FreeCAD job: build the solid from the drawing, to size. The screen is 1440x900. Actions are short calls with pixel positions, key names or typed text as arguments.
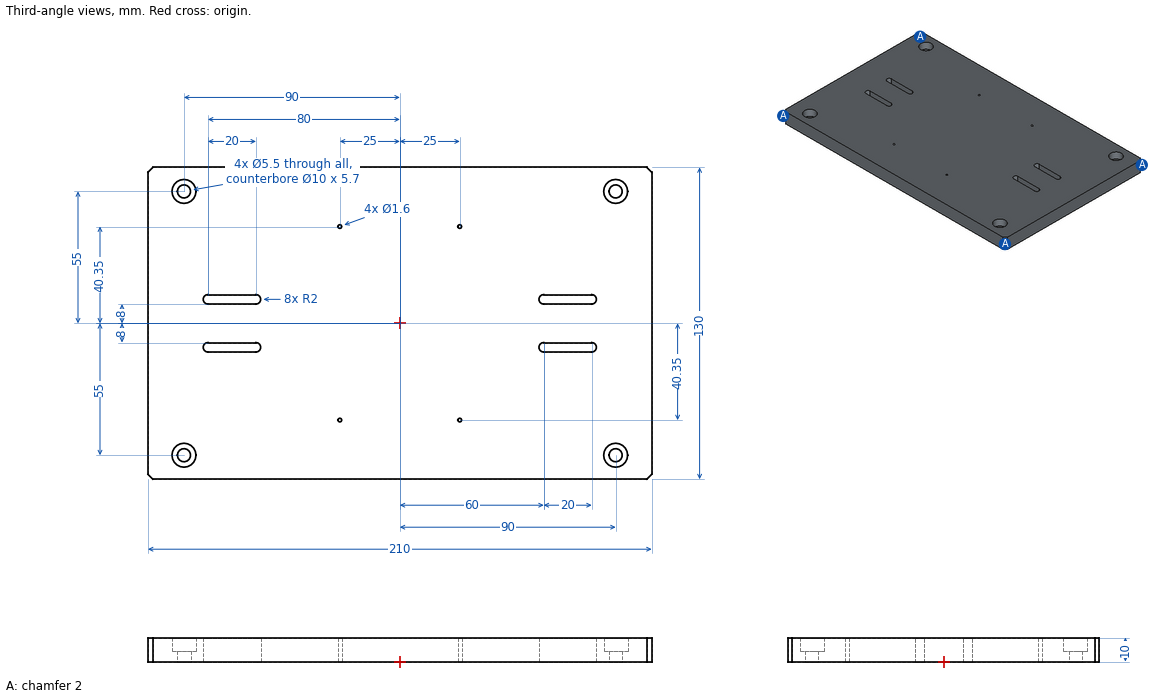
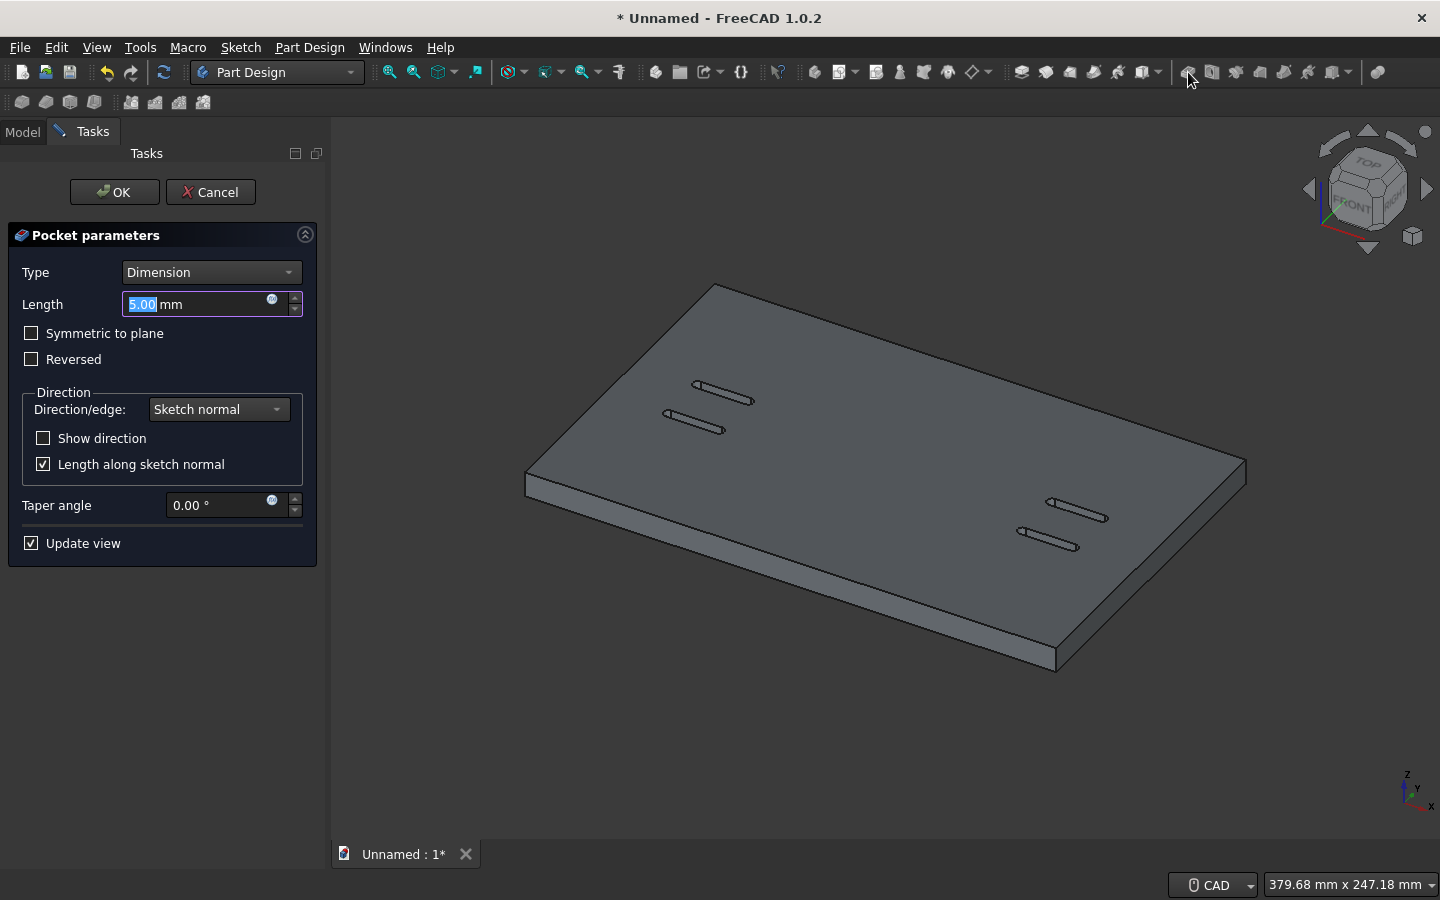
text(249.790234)
key(Tab)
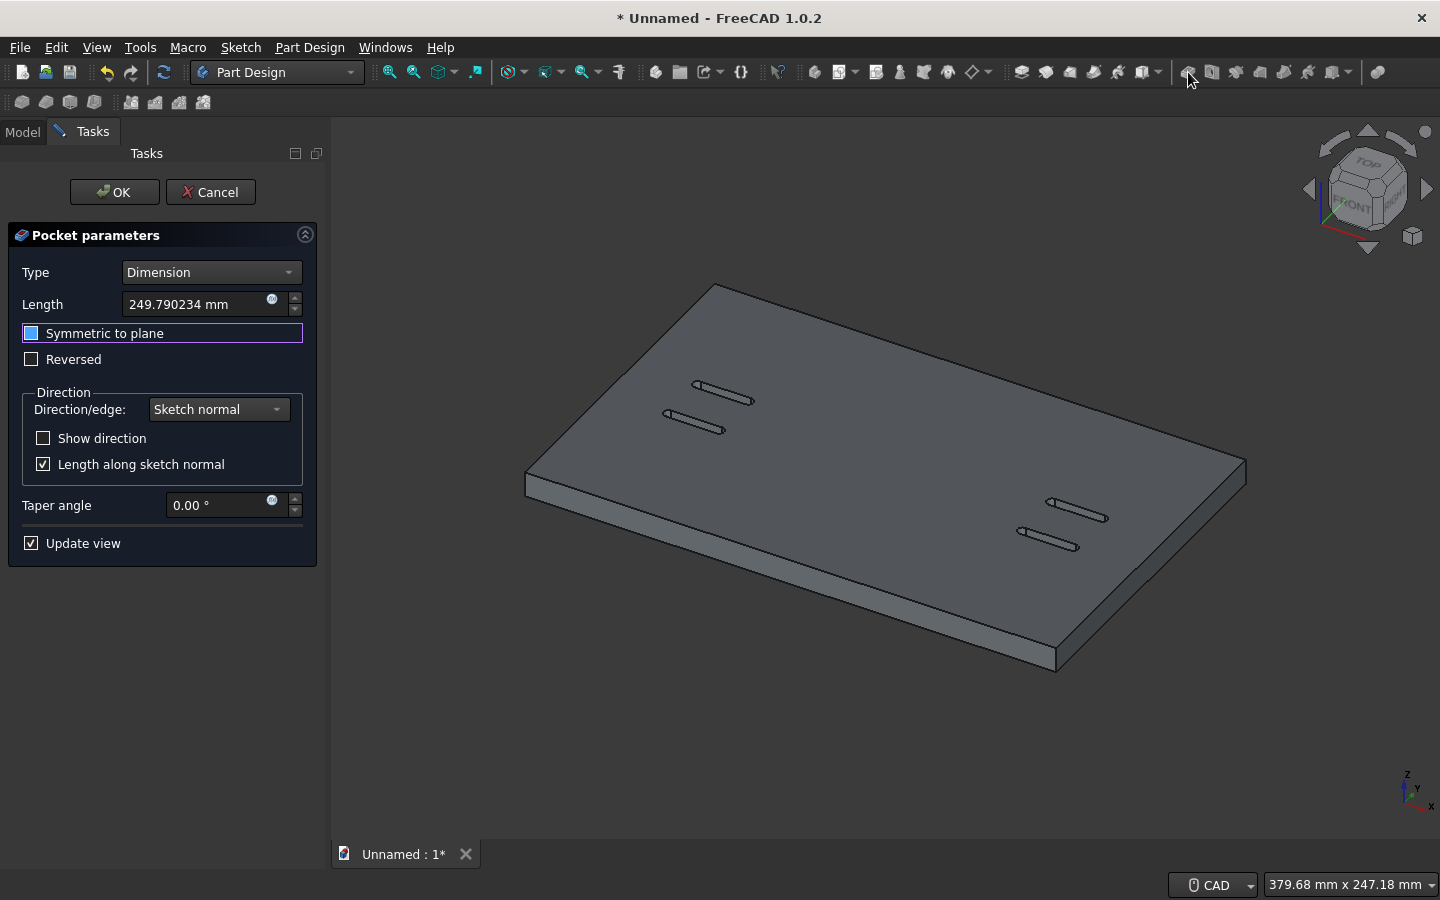
click(30, 333)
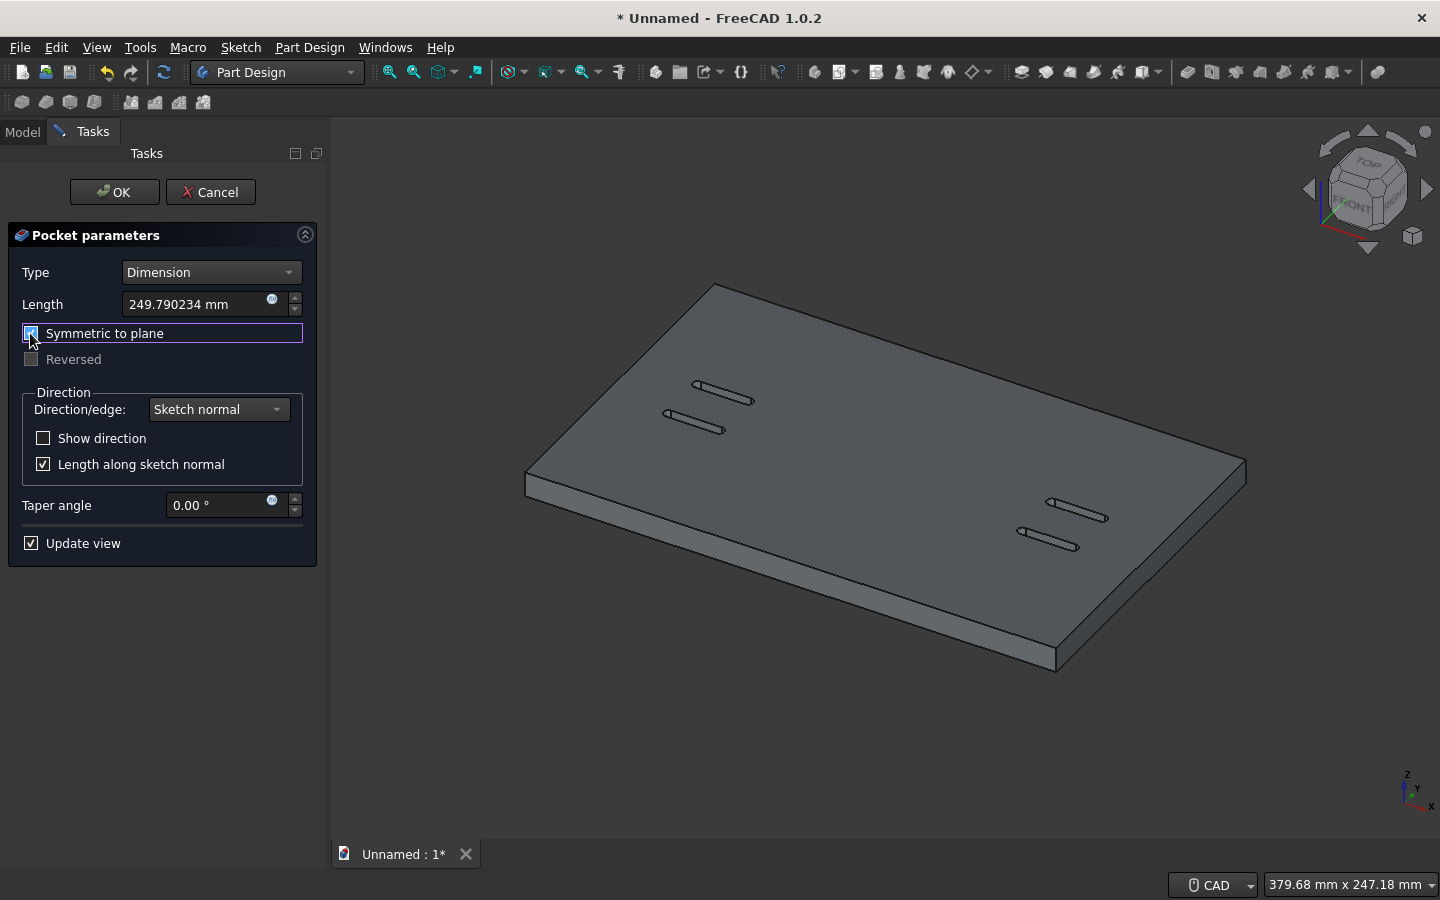
click(115, 192)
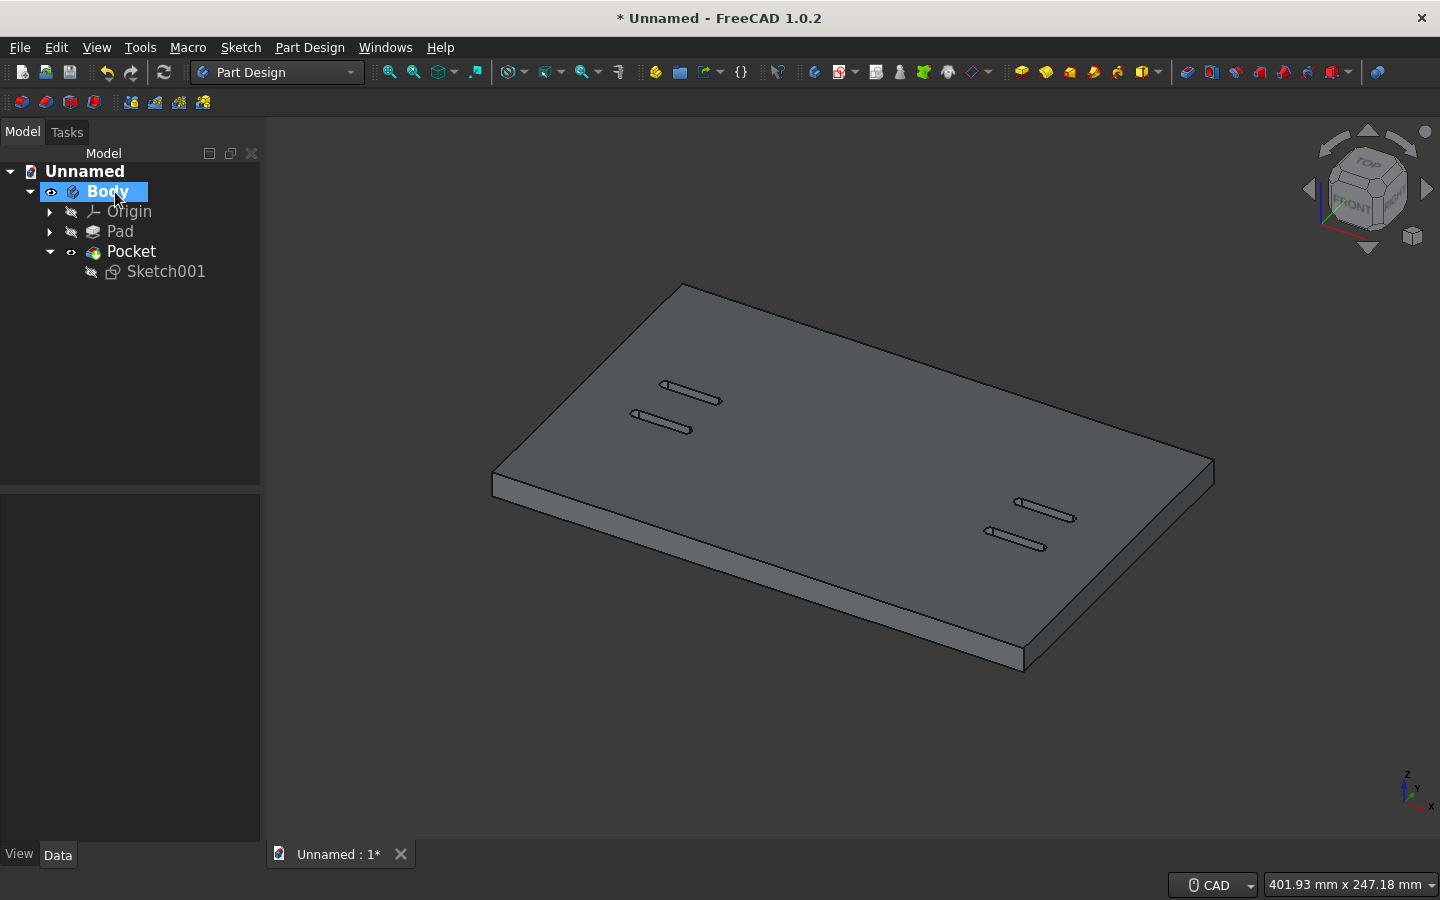
click(853, 465)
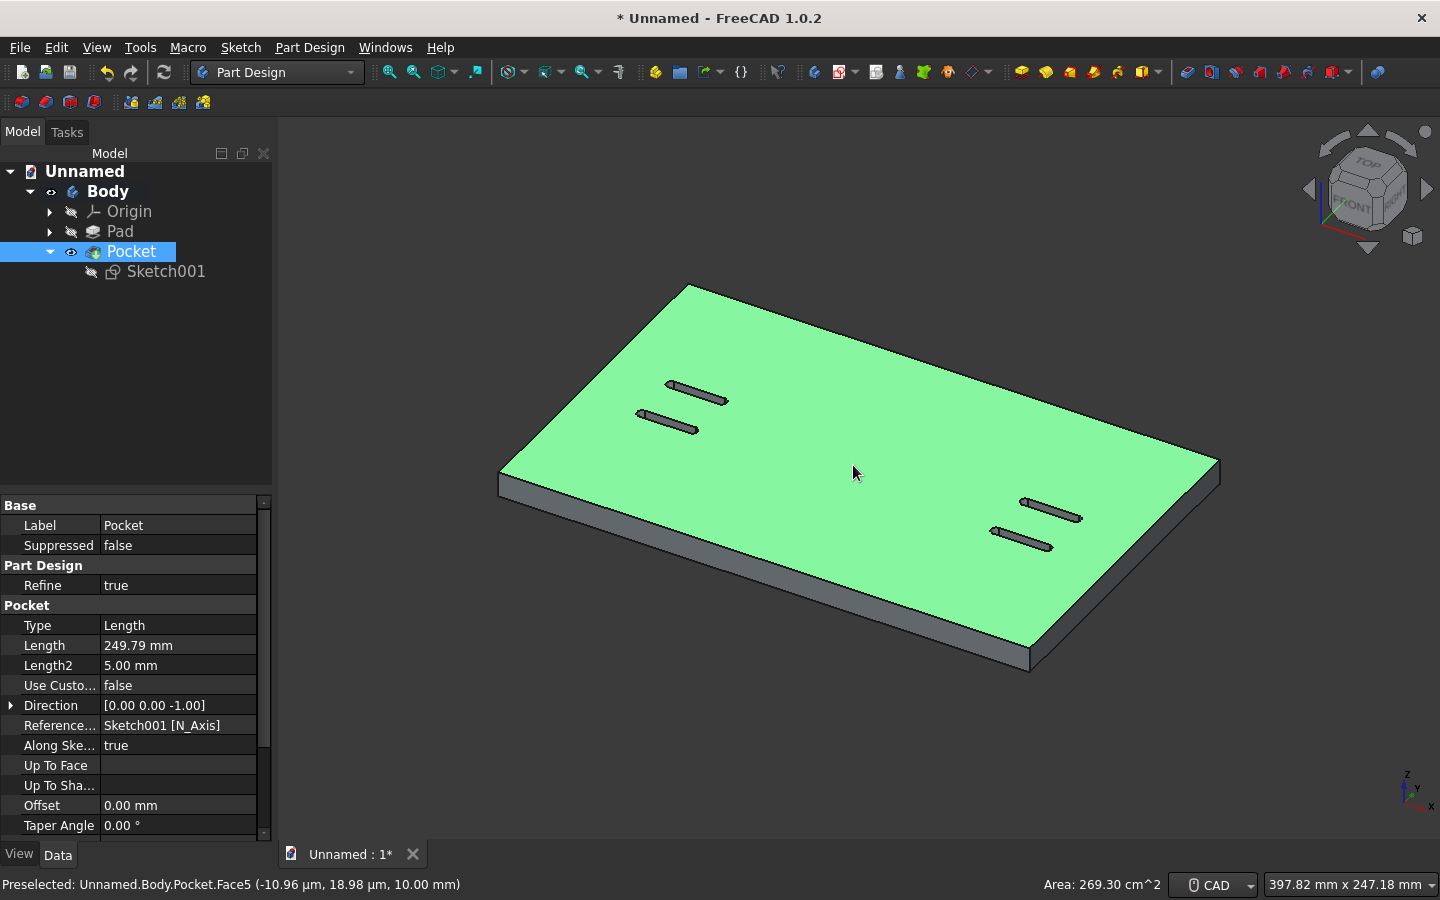
click(840, 72)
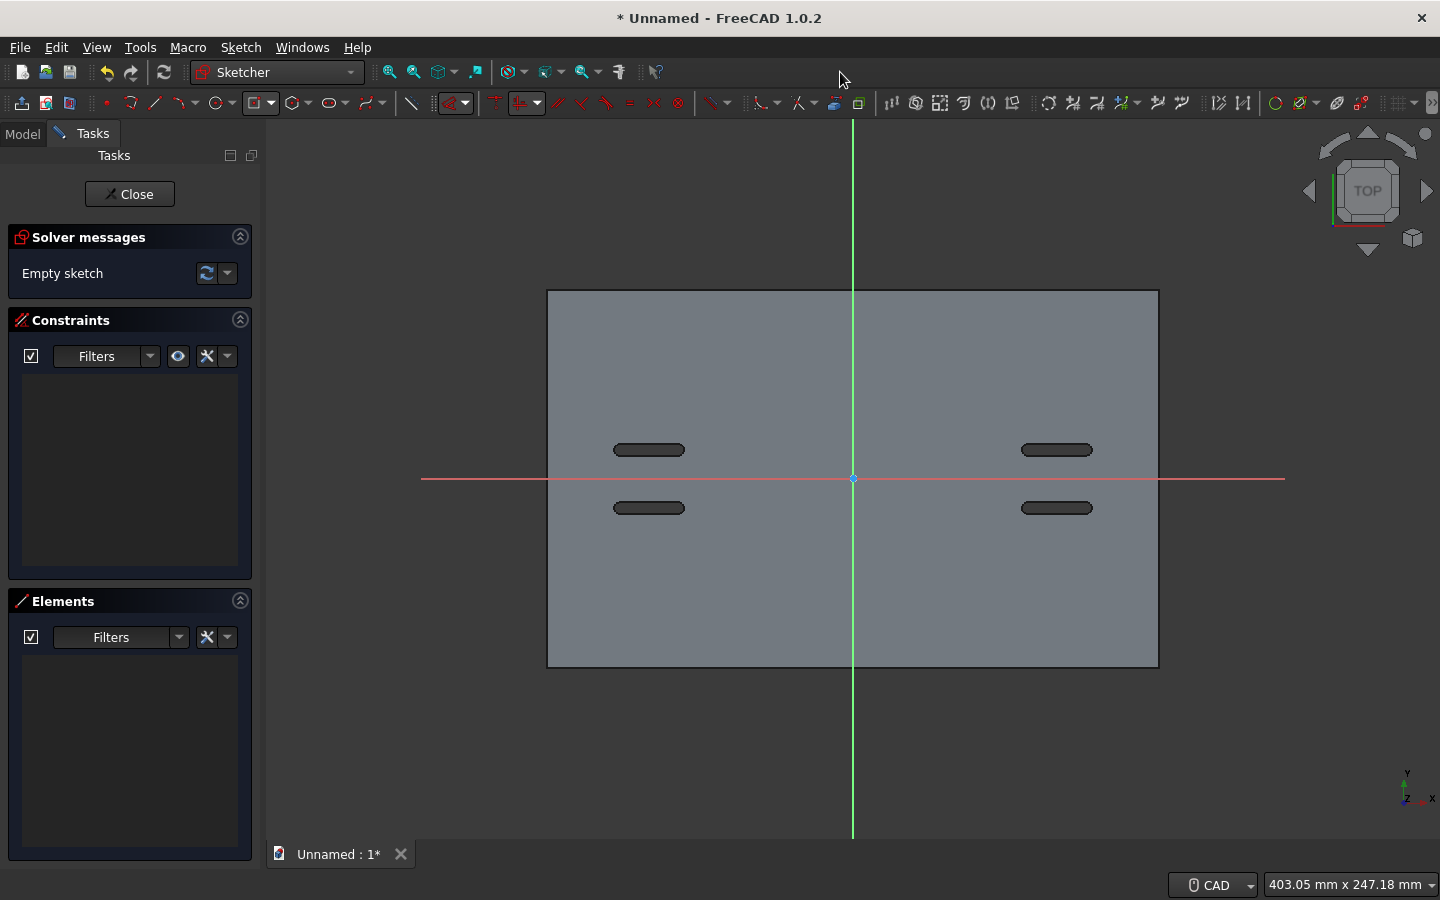
click(216, 104)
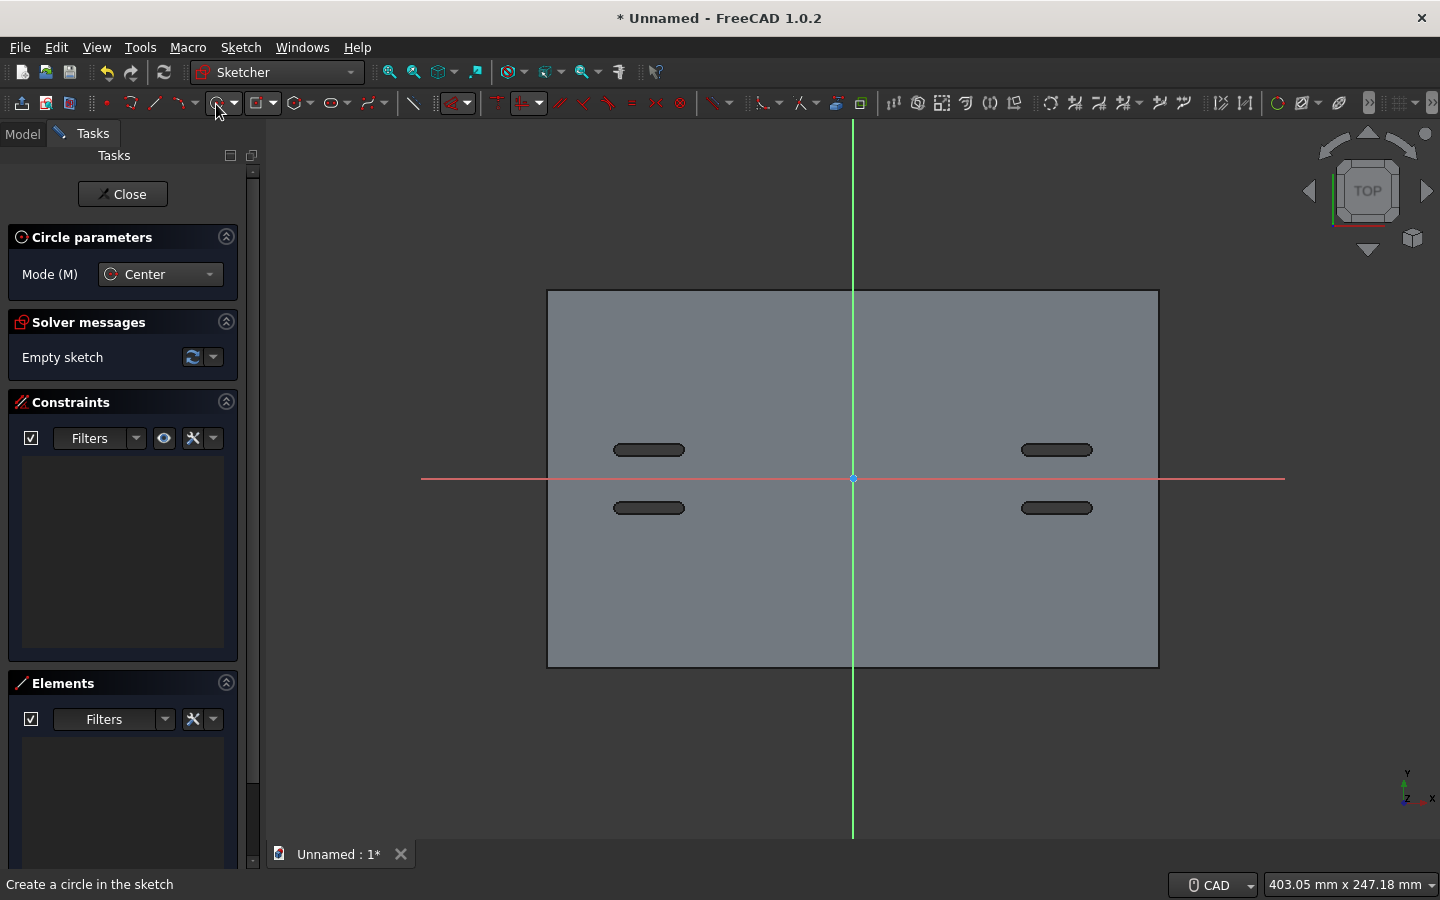
scroll(591, 319, up, 6)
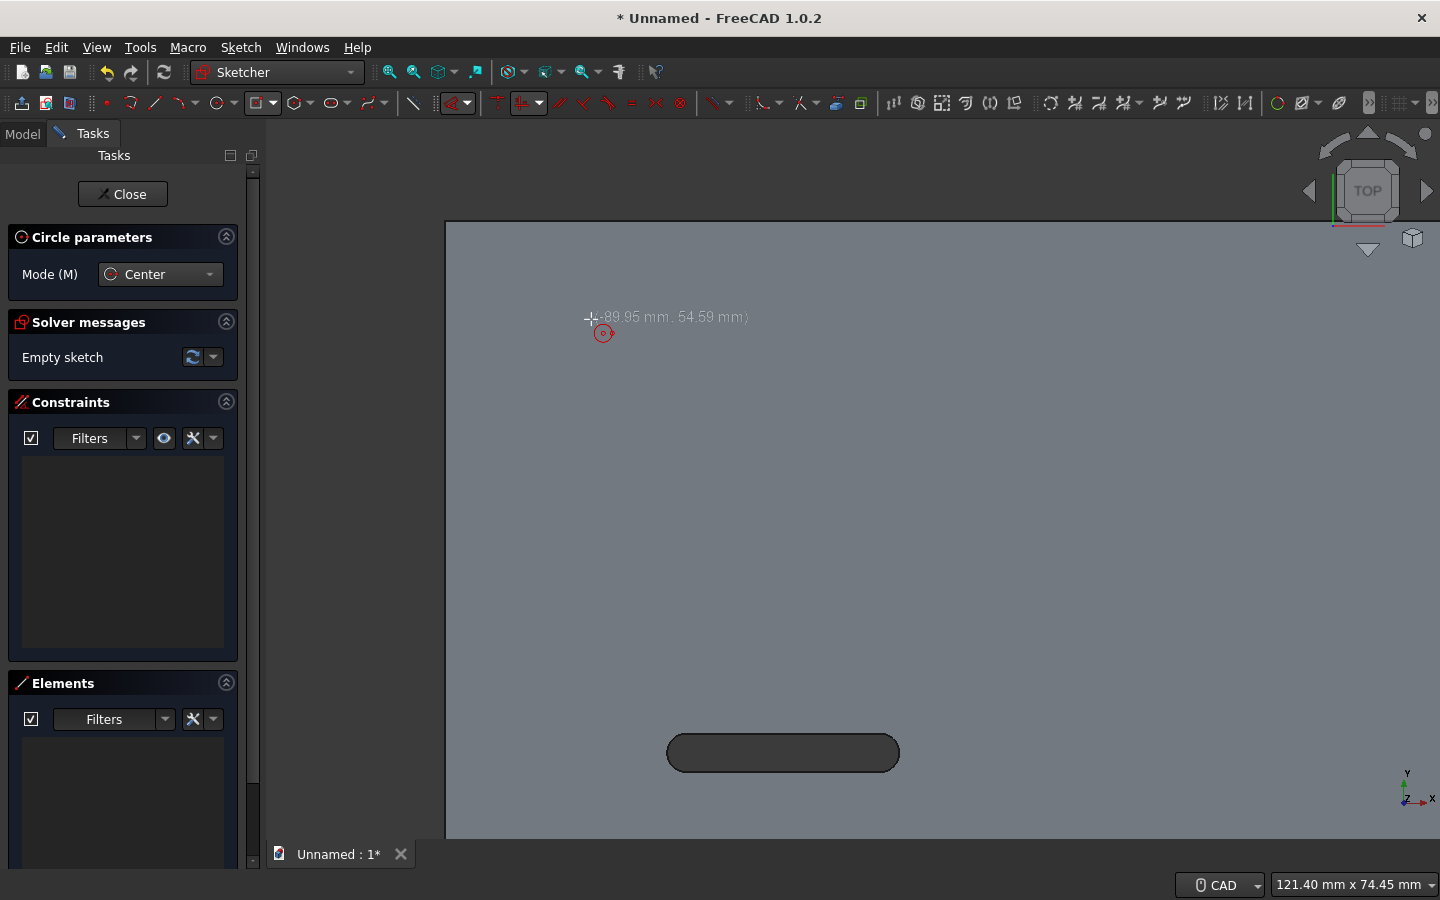
click(590, 318)
move(609, 299)